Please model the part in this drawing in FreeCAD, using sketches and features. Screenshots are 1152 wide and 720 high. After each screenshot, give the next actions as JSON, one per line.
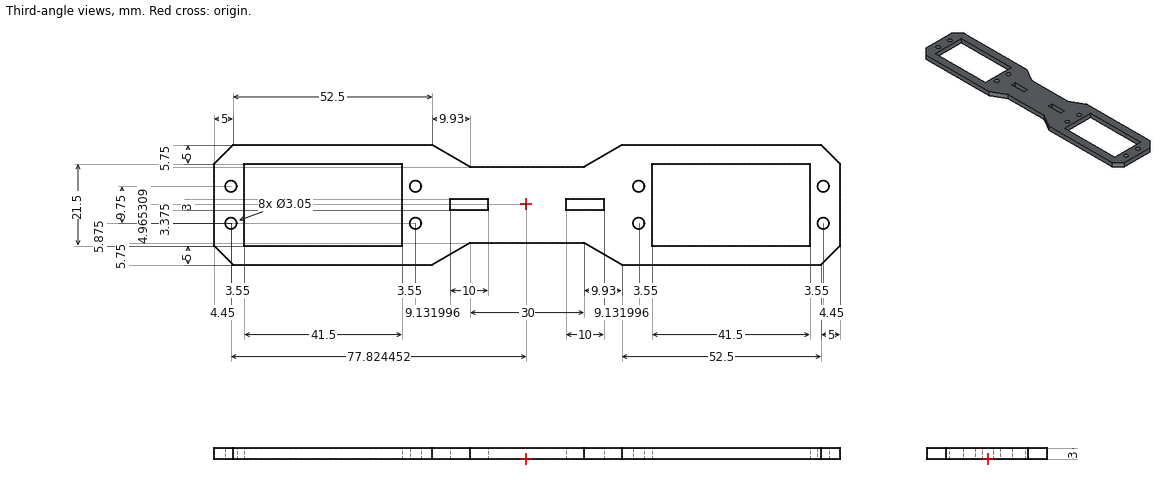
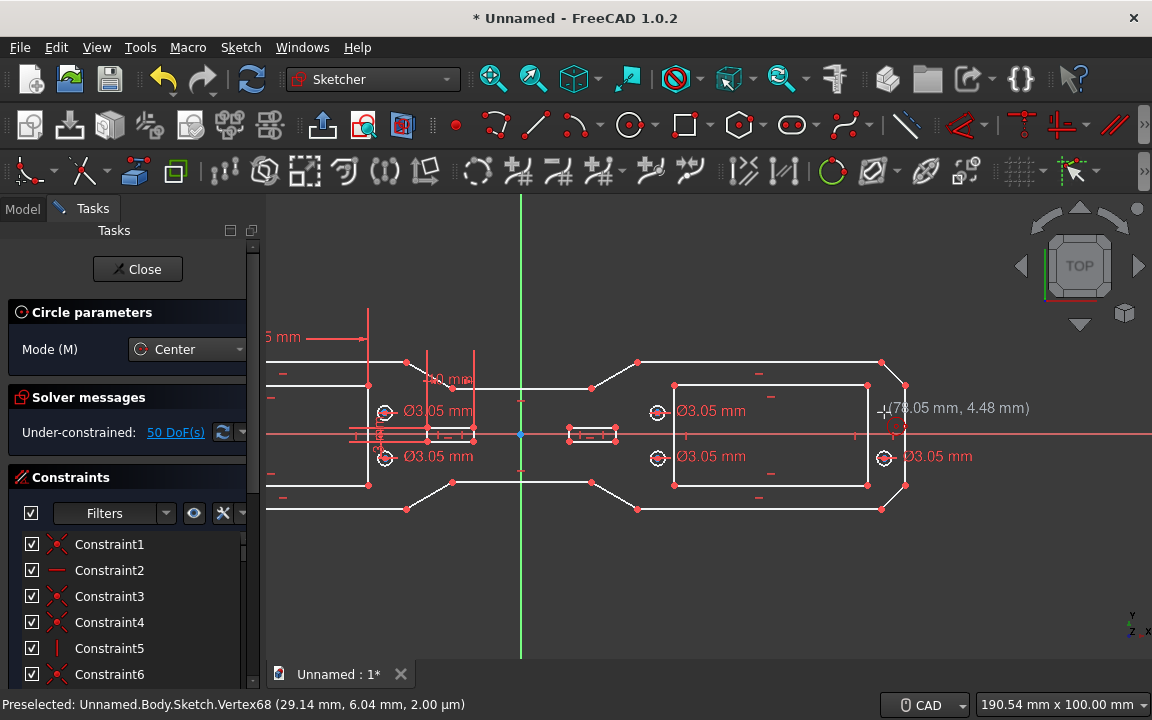
{"action": "left_click", "coordinate": [884, 412]}
{"action": "mouse_move", "coordinate": [889, 407]}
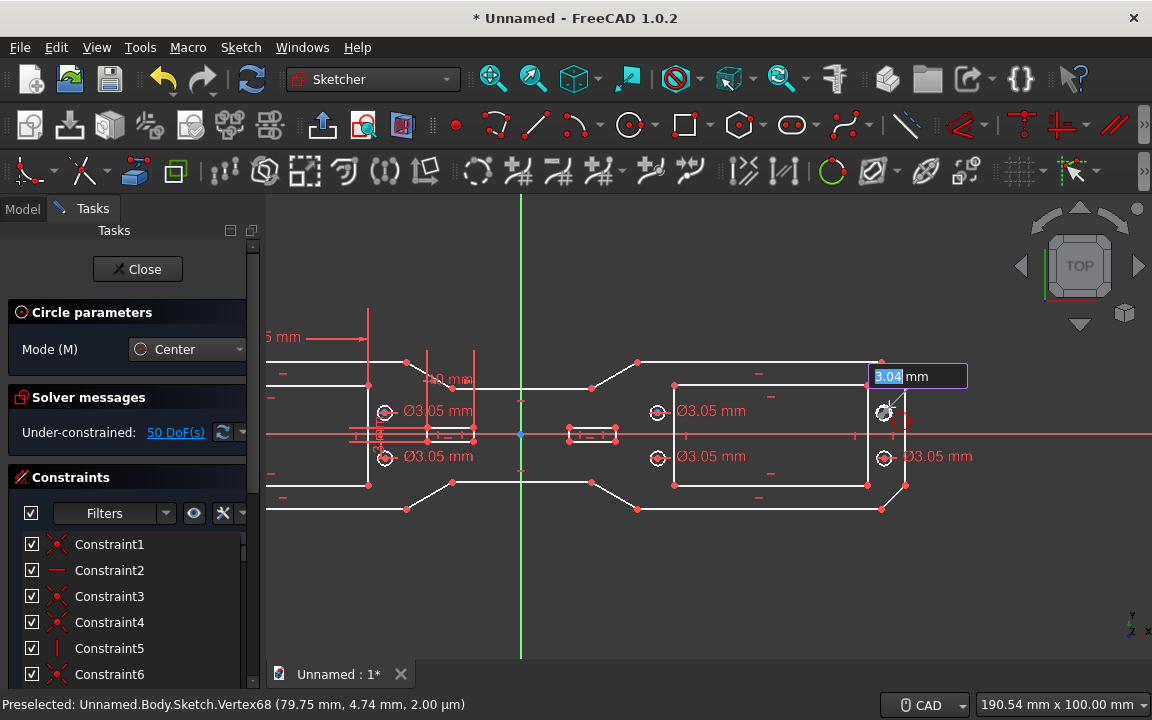
{"action": "type", "text": "3.05"}
{"action": "key", "text": "Return"}
{"action": "key", "text": "Escape"}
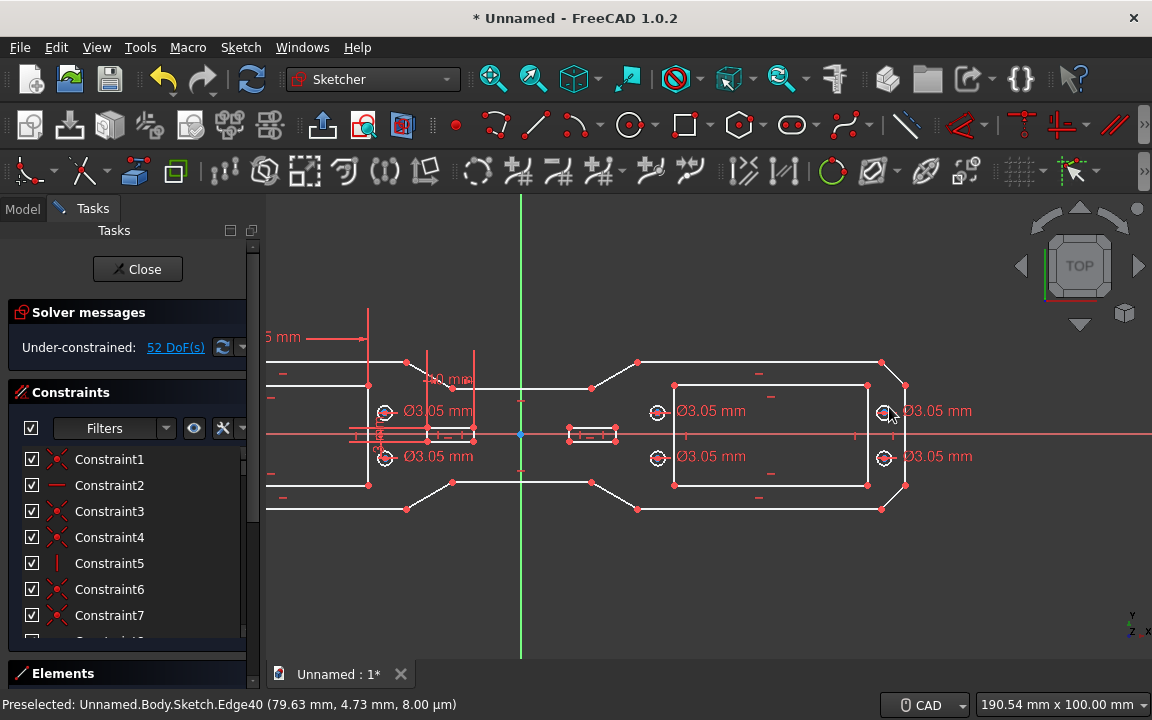
{"action": "left_click", "coordinate": [960, 126]}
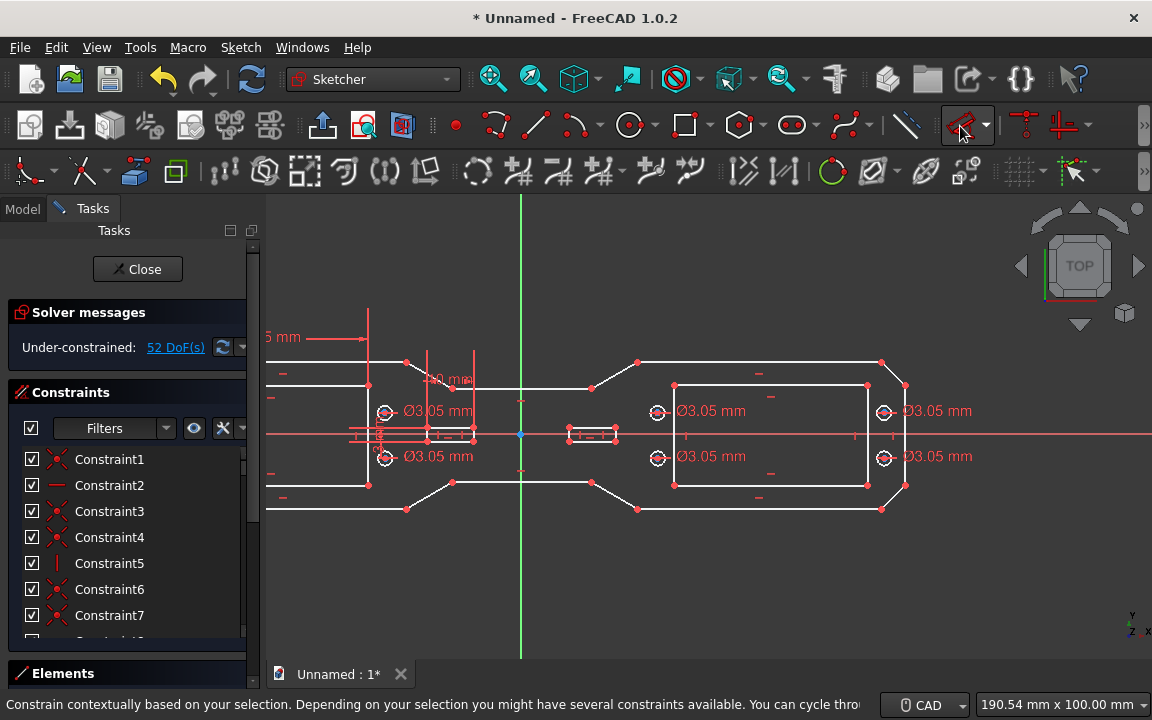
{"action": "scroll", "coordinate": [569, 435], "scroll_direction": "up", "scroll_amount": 6}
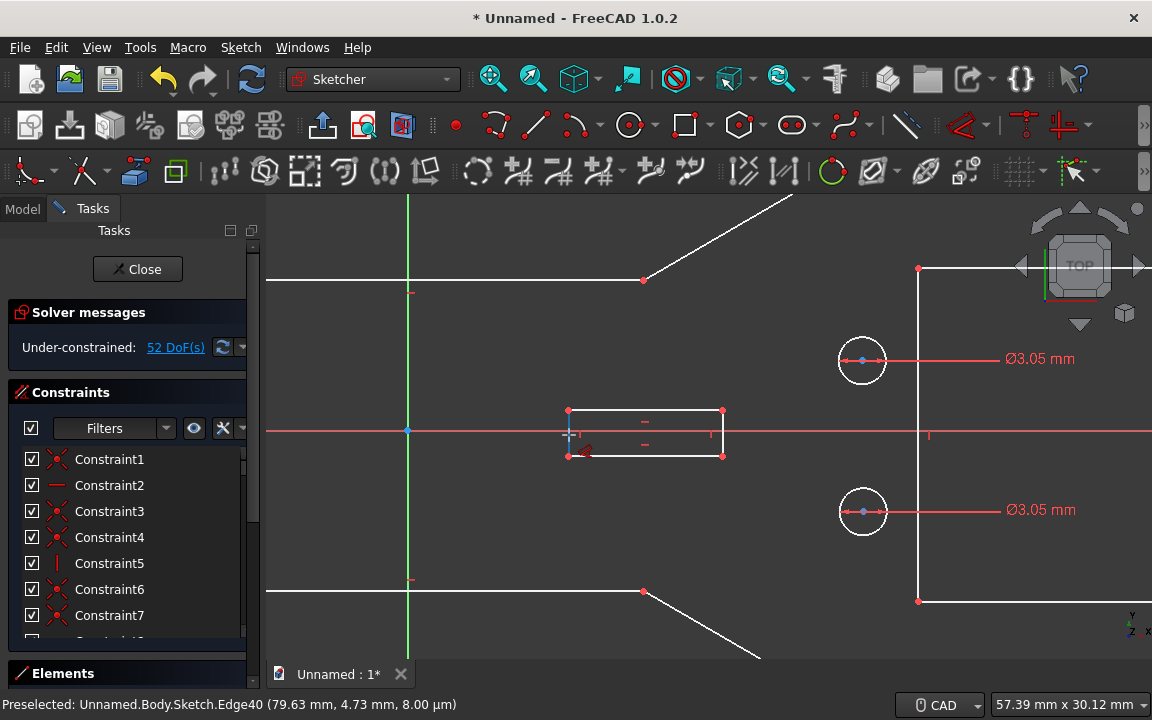
{"action": "left_click", "coordinate": [569, 433]}
{"action": "left_click", "coordinate": [535, 444]}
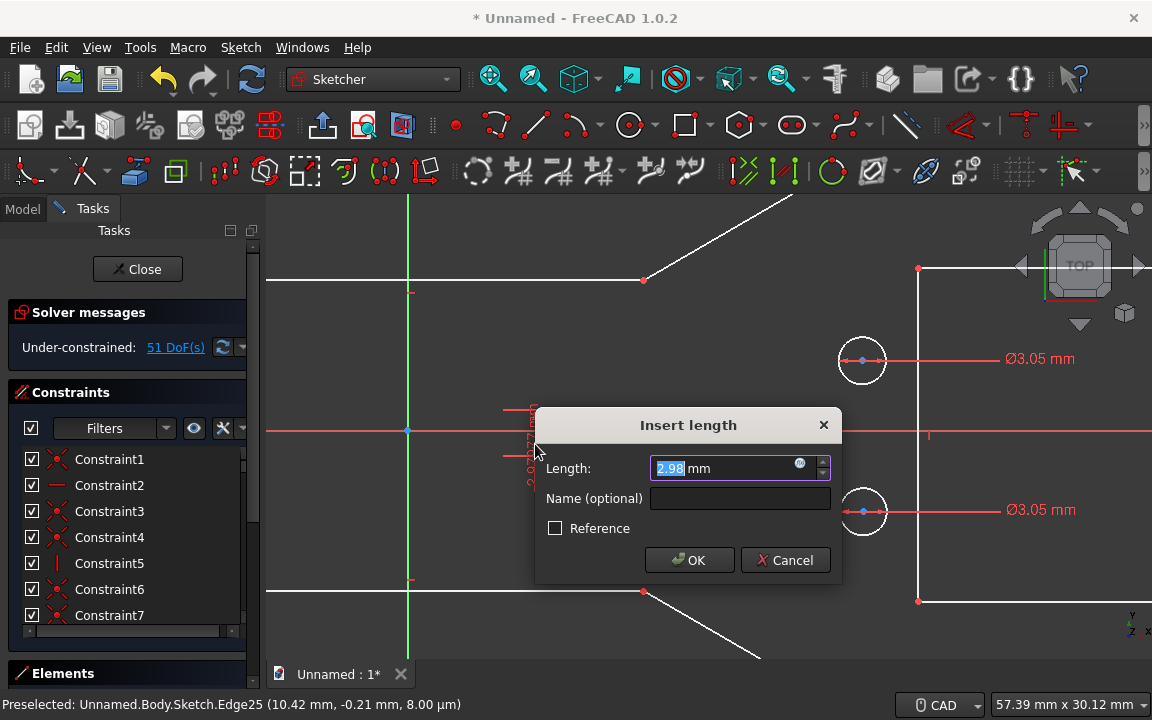
{"action": "type", "text": "3"}
{"action": "key", "text": "Return"}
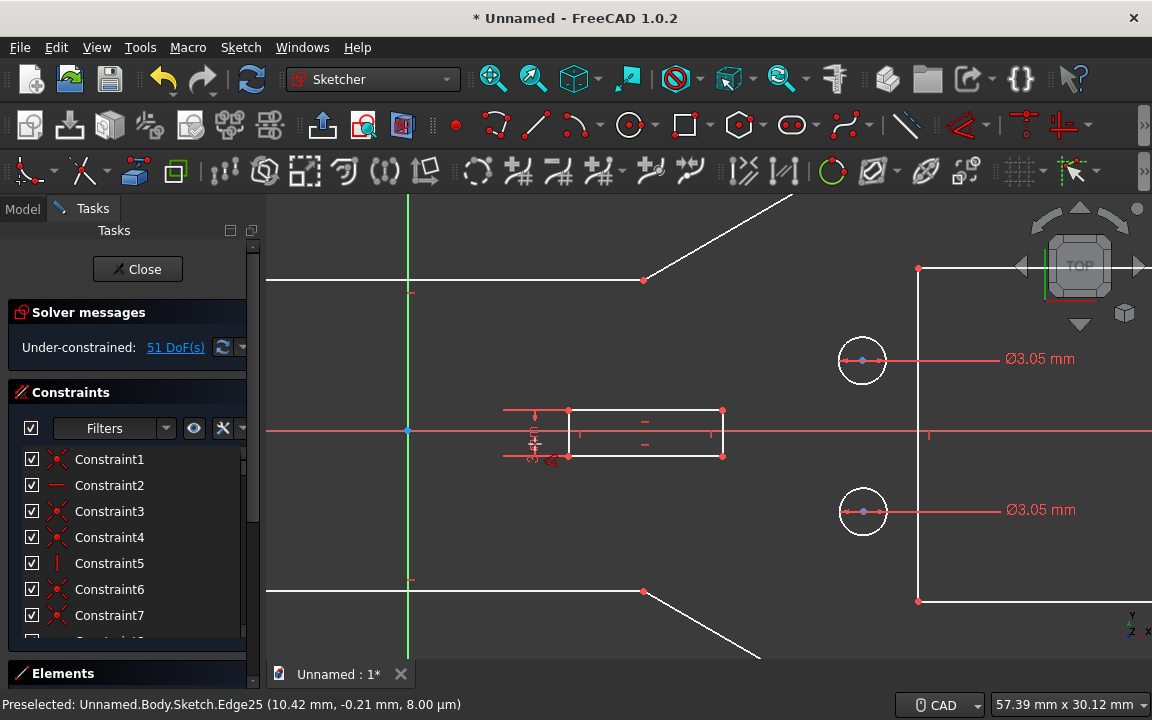
{"action": "scroll", "coordinate": [699, 425], "scroll_direction": "down", "scroll_amount": 8}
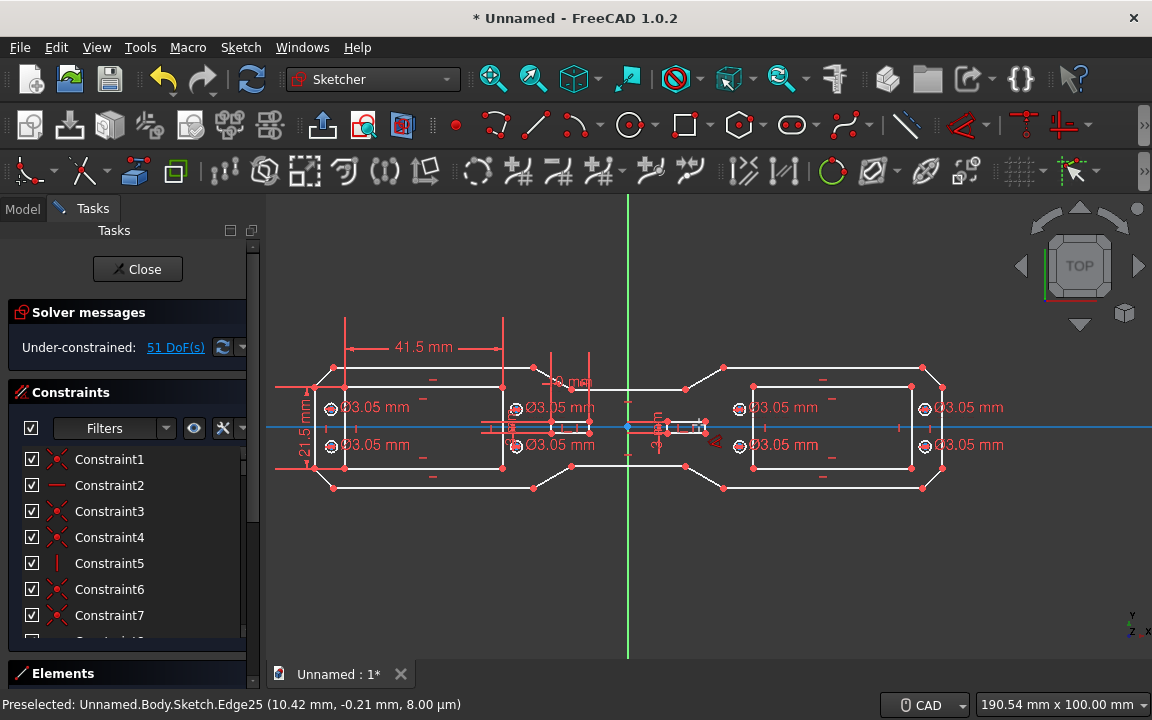
{"action": "left_click", "coordinate": [623, 459]}
{"action": "left_click", "coordinate": [620, 493]}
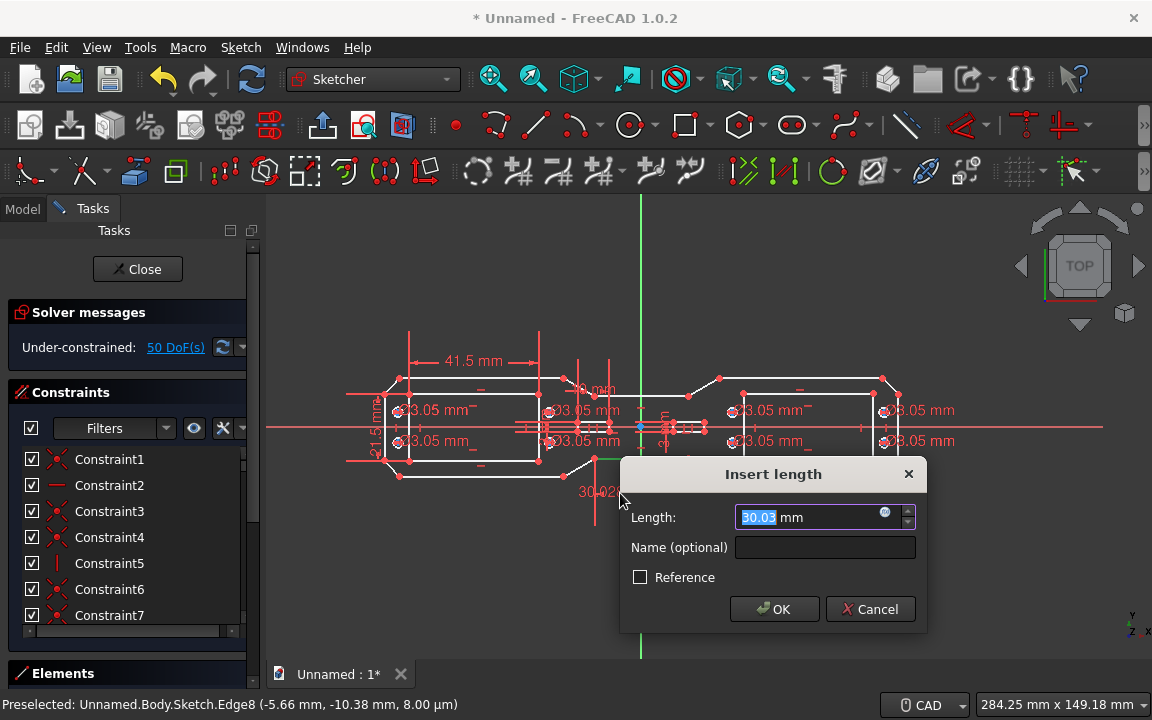
{"action": "type", "text": "30"}
{"action": "key", "text": "Return"}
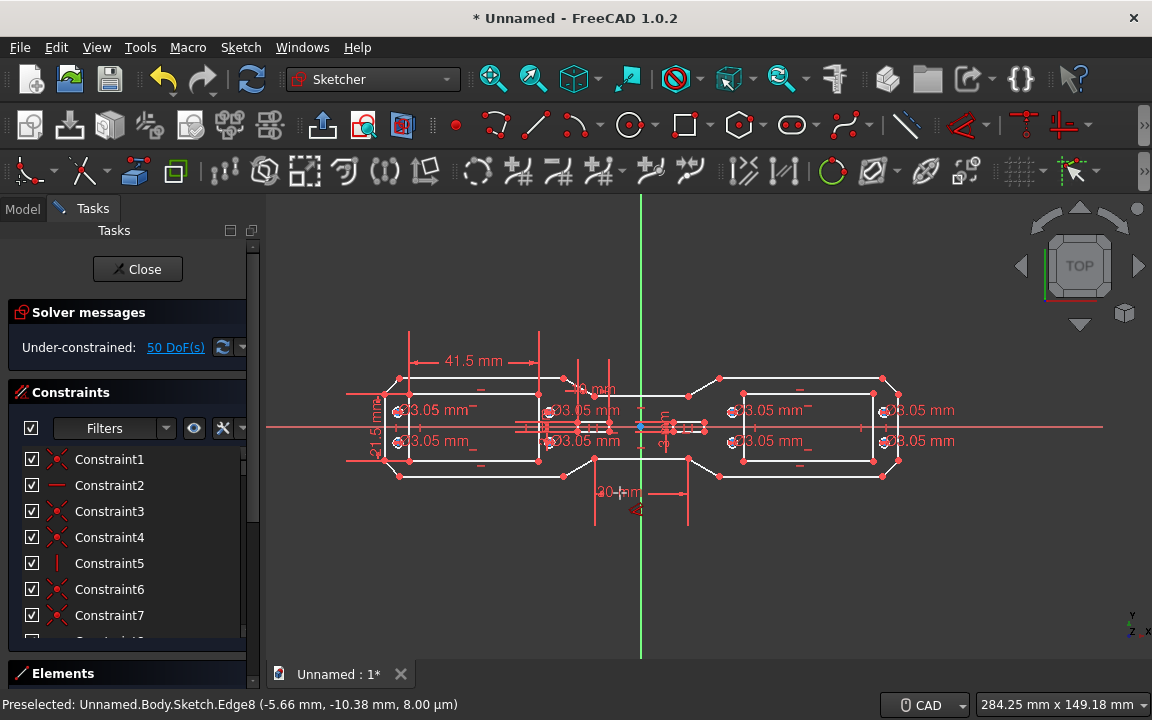
{"action": "left_click", "coordinate": [660, 396]}
{"action": "left_click", "coordinate": [620, 362]}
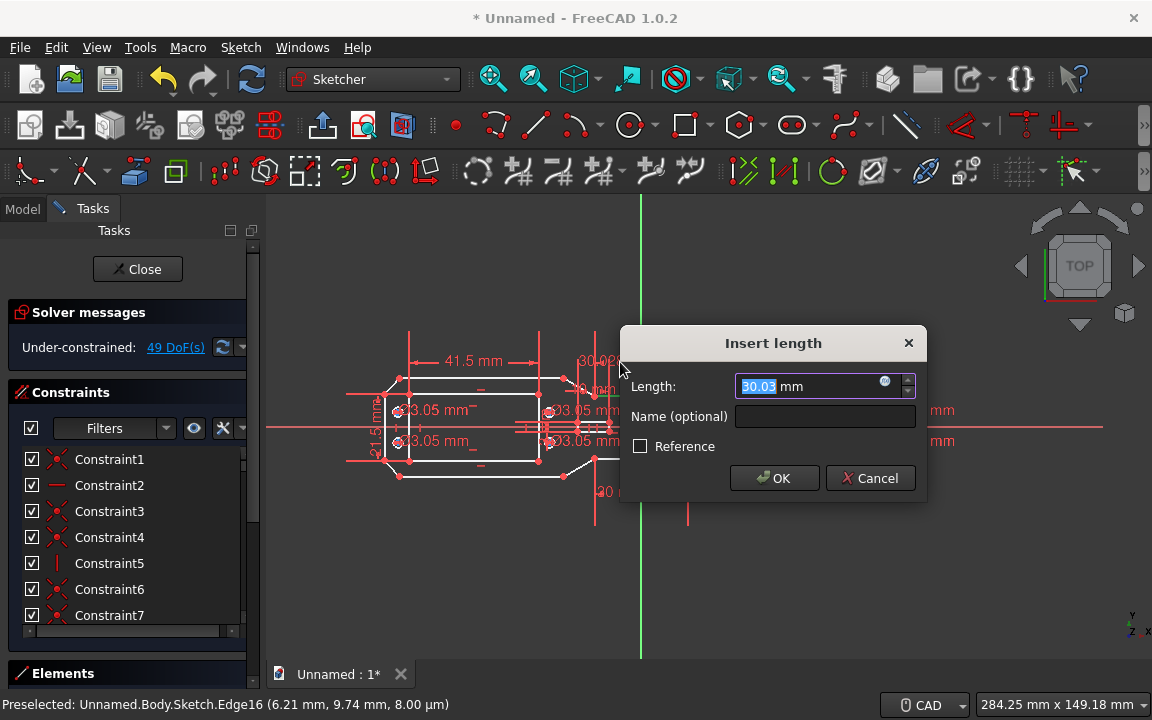
{"action": "type", "text": "30"}
{"action": "key", "text": "Return"}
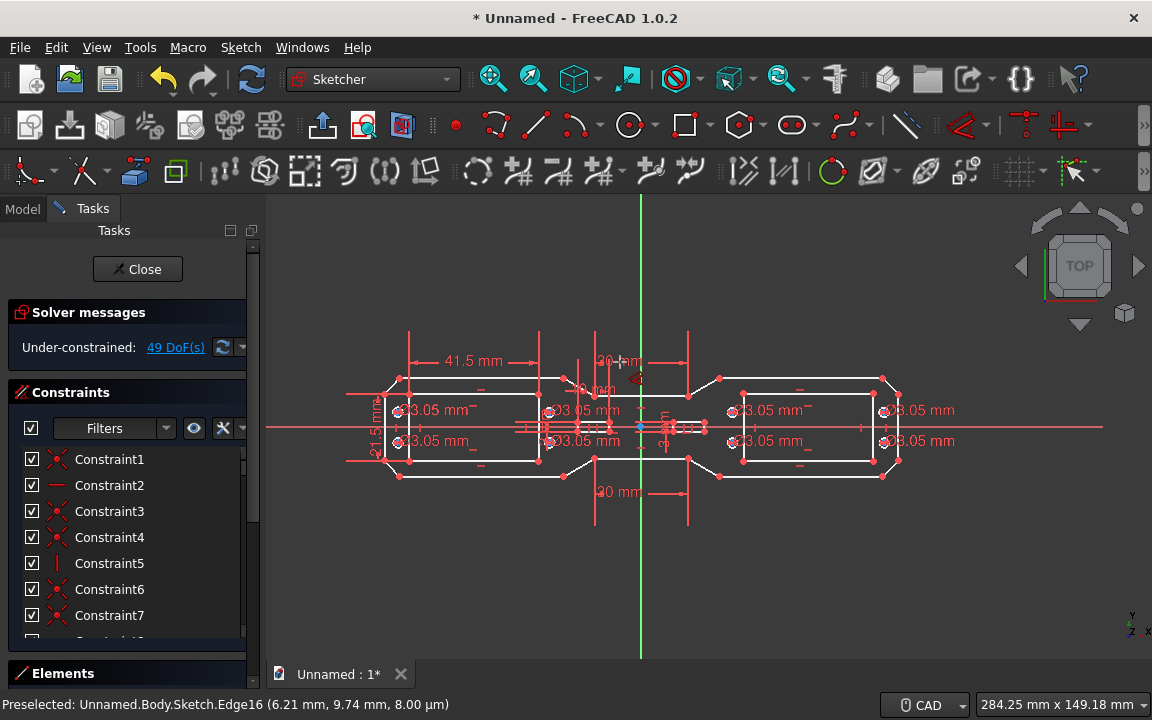
{"action": "scroll", "coordinate": [682, 432], "scroll_direction": "up", "scroll_amount": 5}